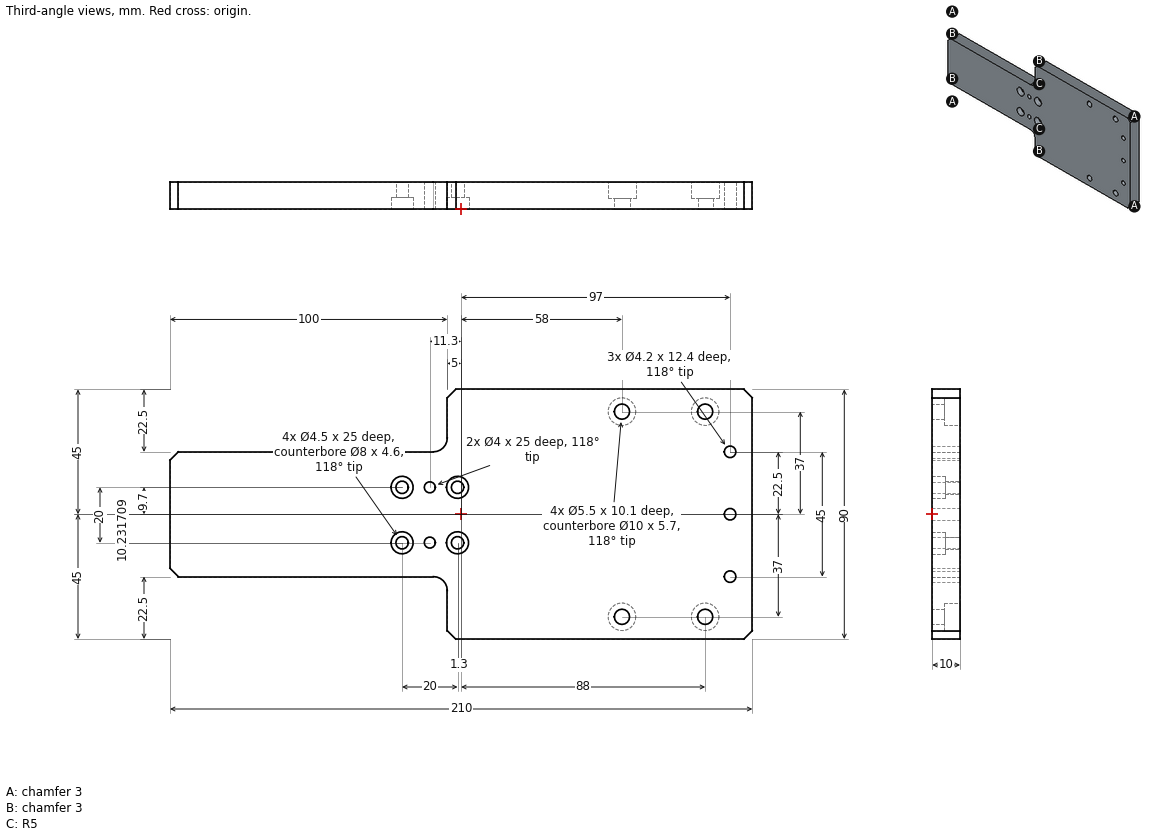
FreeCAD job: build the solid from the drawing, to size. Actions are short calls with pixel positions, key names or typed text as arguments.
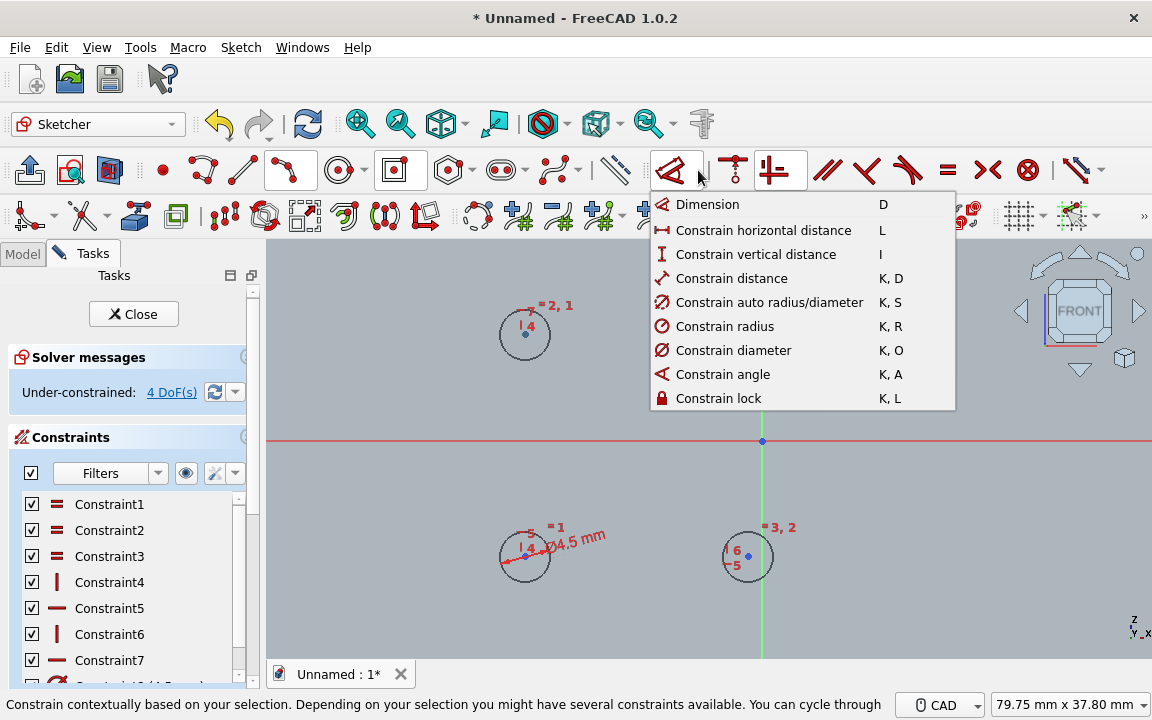
click(803, 254)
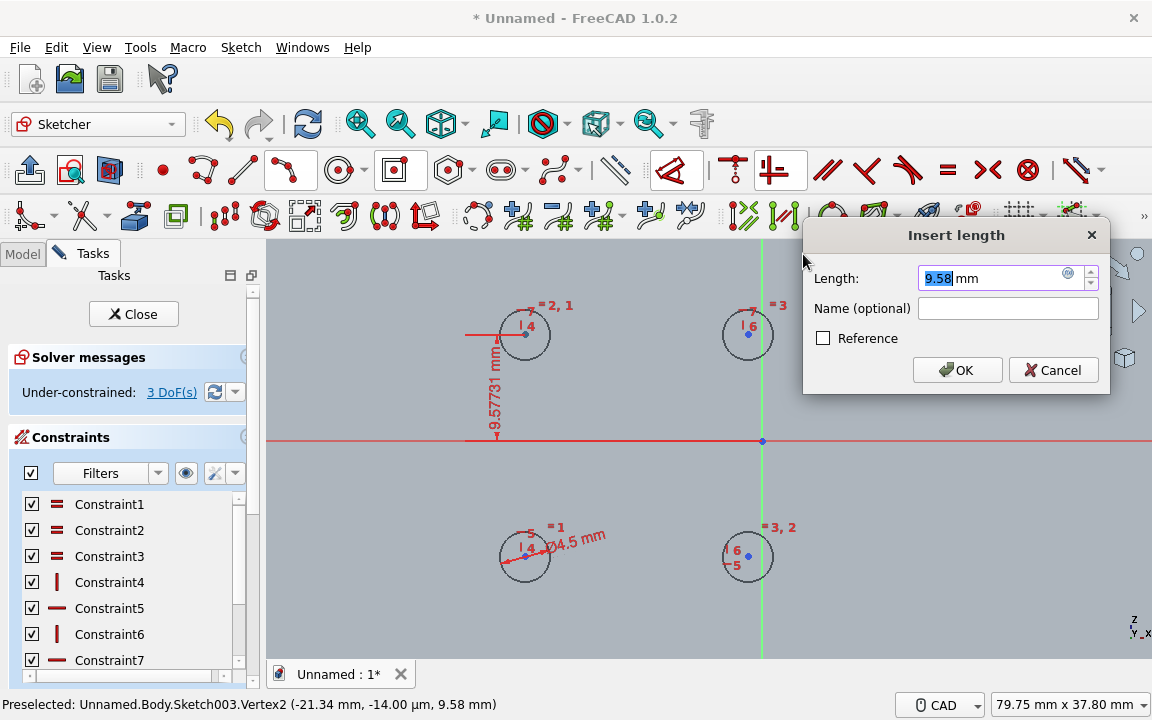
text(9.7)
key(Return)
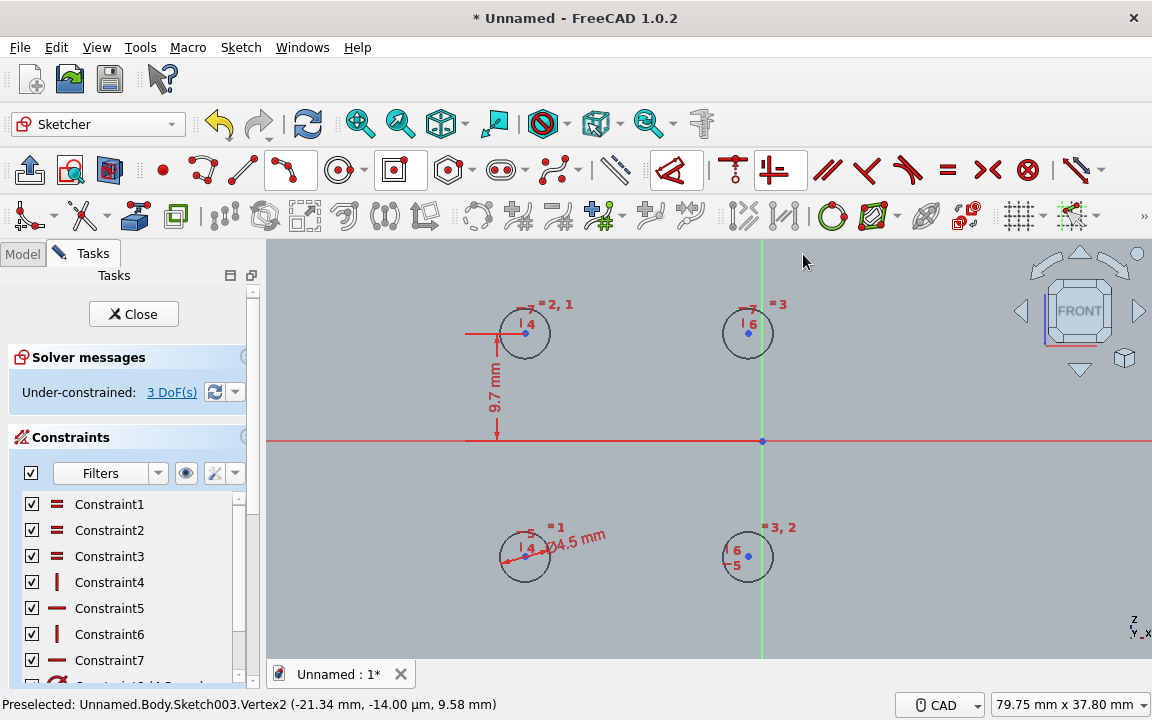
scroll(748, 557, up, 6)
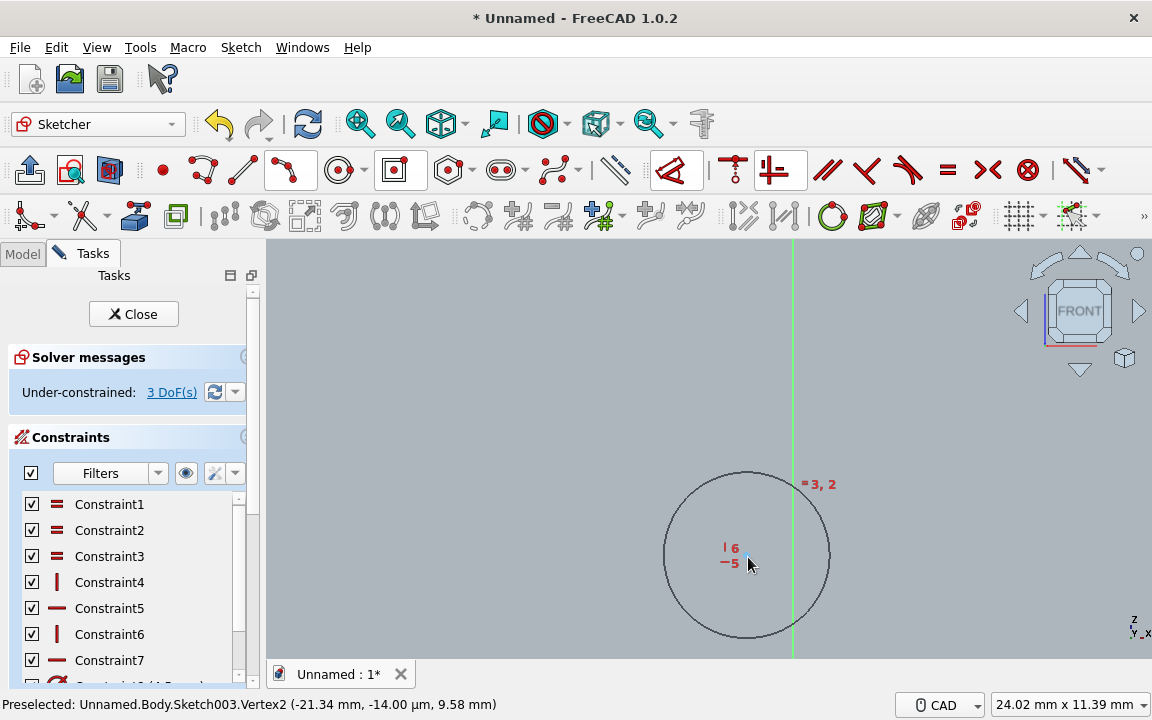
click(747, 555)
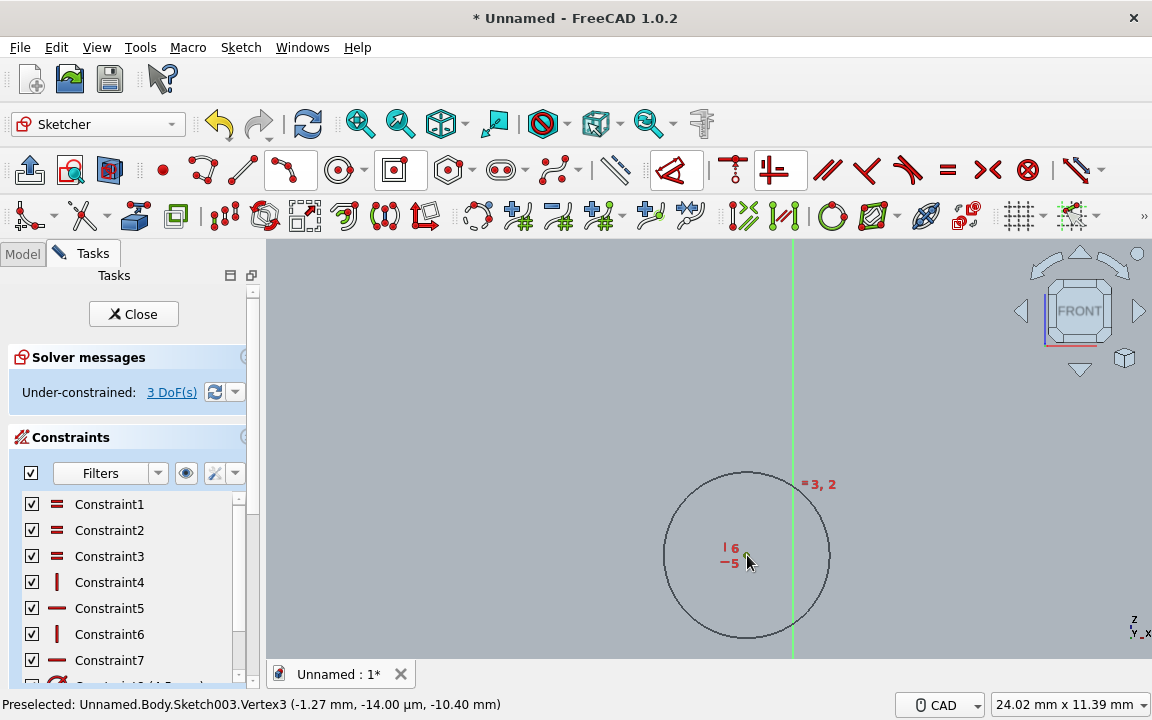
click(698, 170)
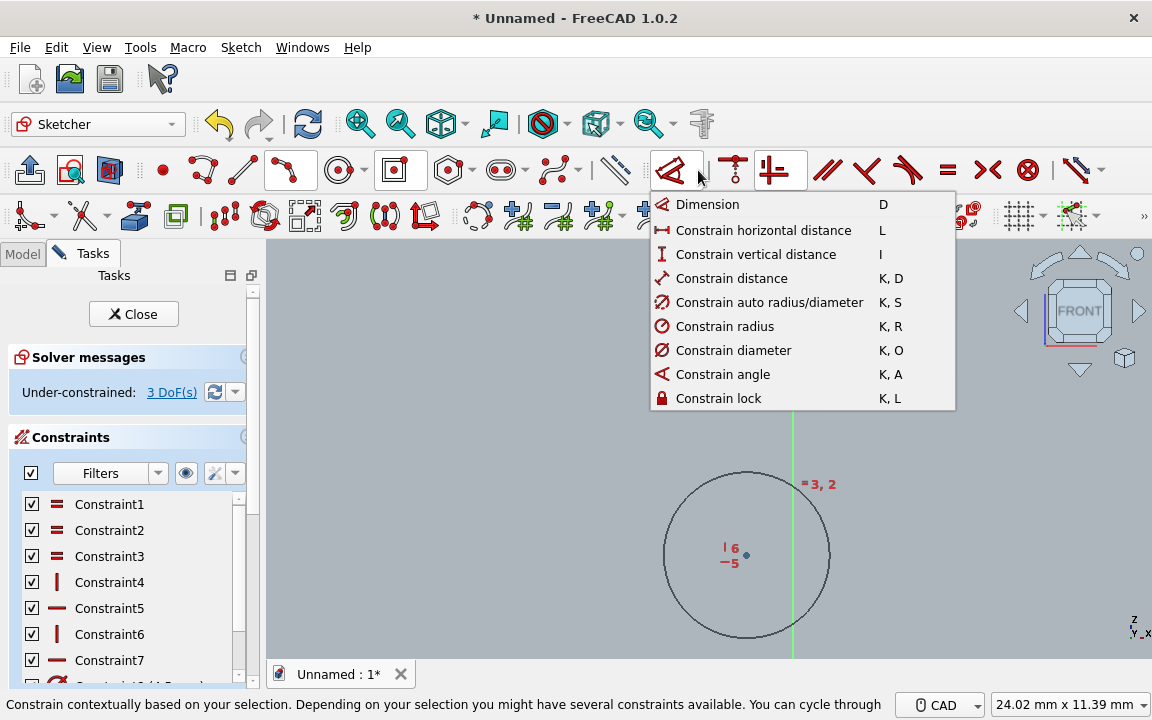
click(803, 230)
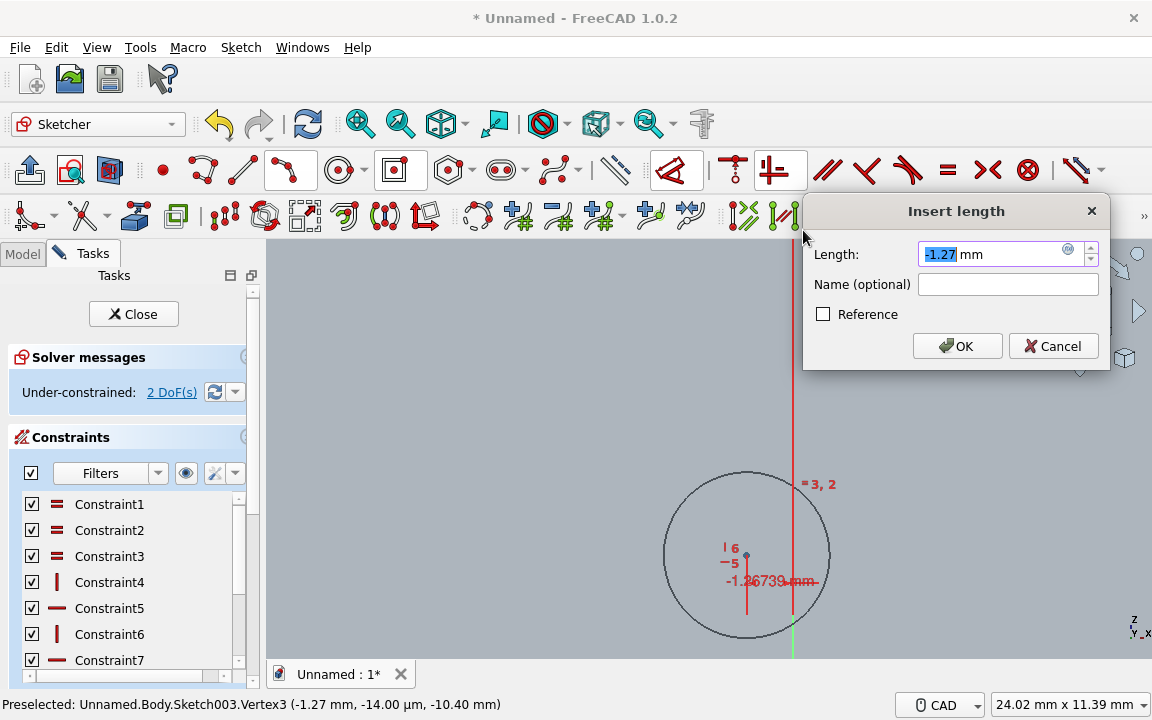
text(-1.3)
key(Return)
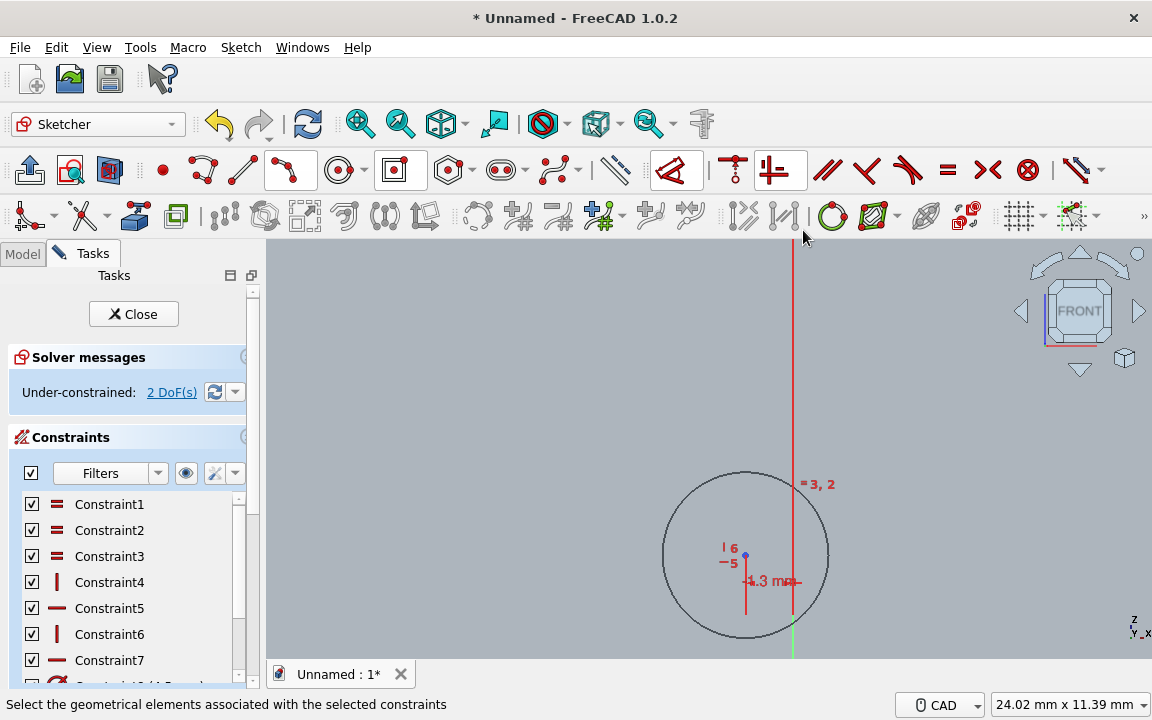
scroll(754, 564, down, 6)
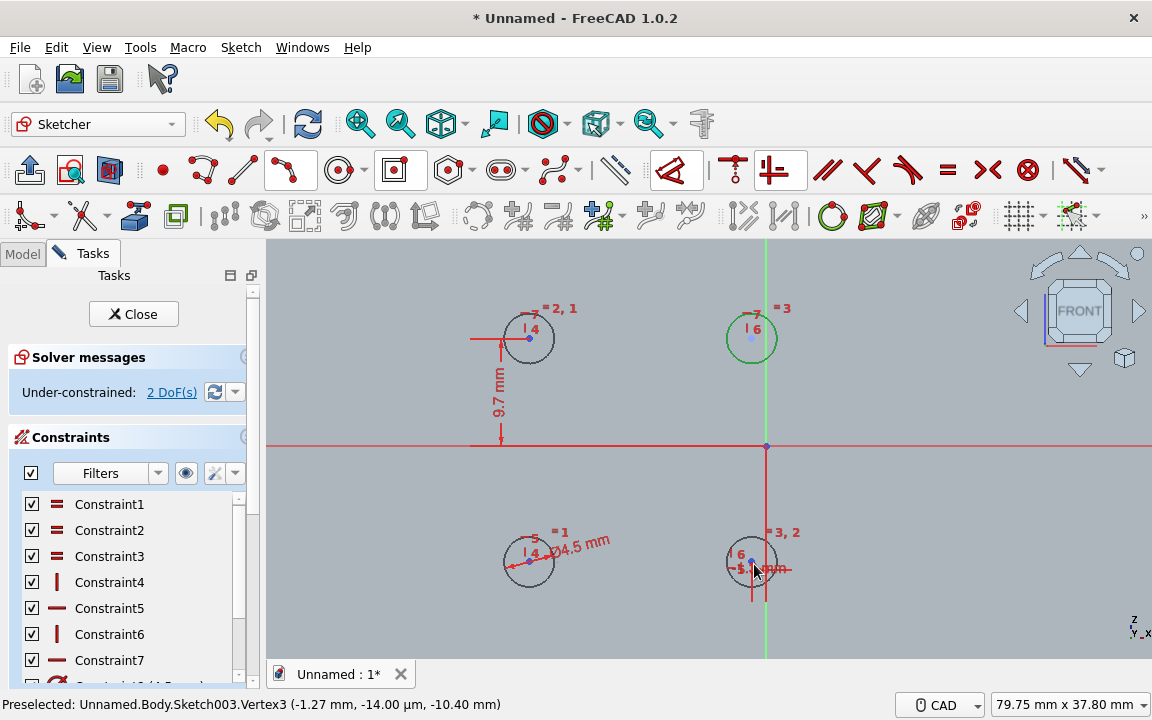
click(529, 562)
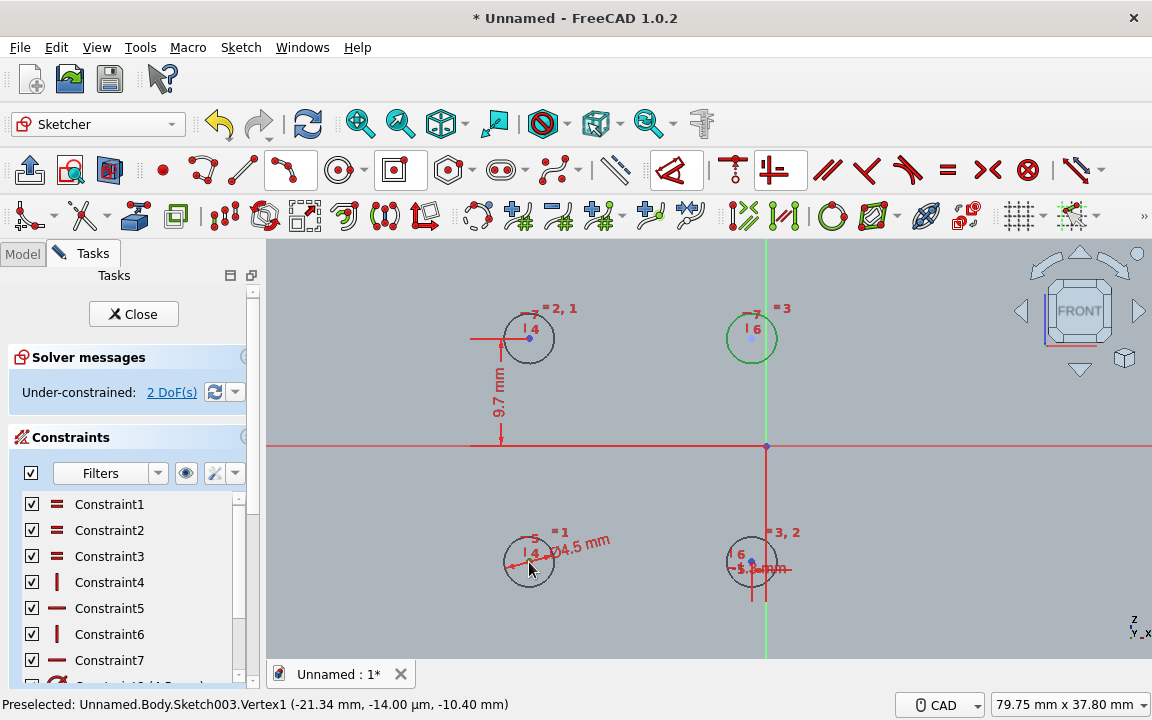
click(529, 339)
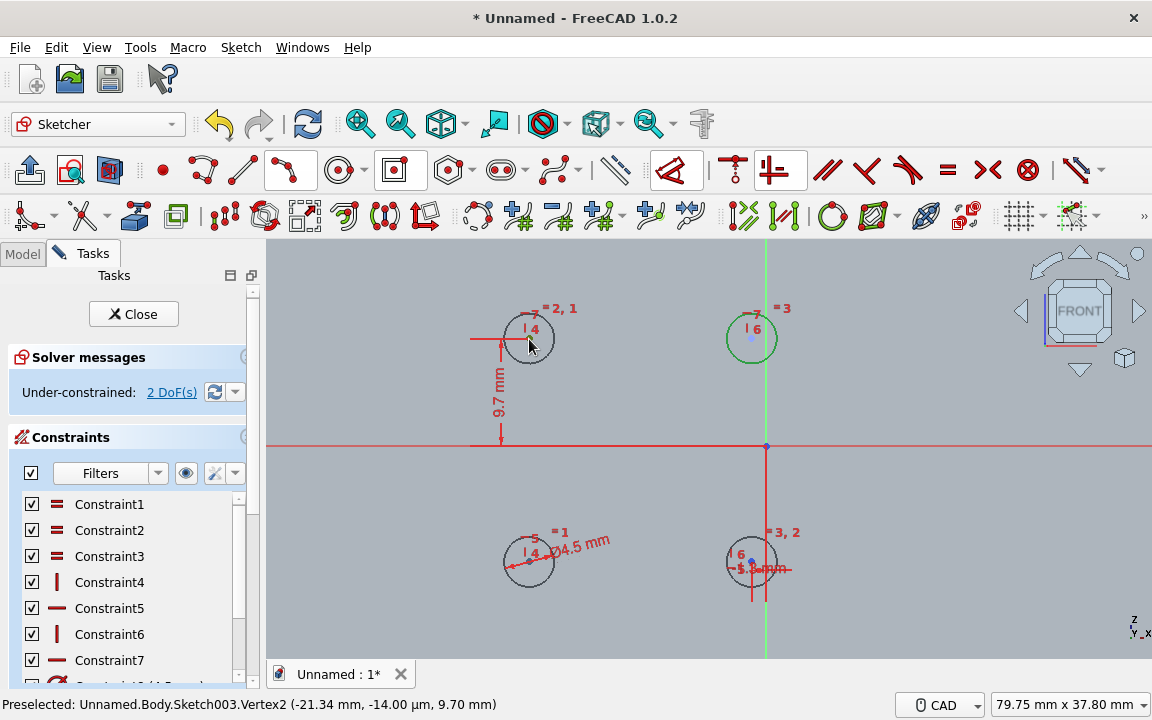
key(i)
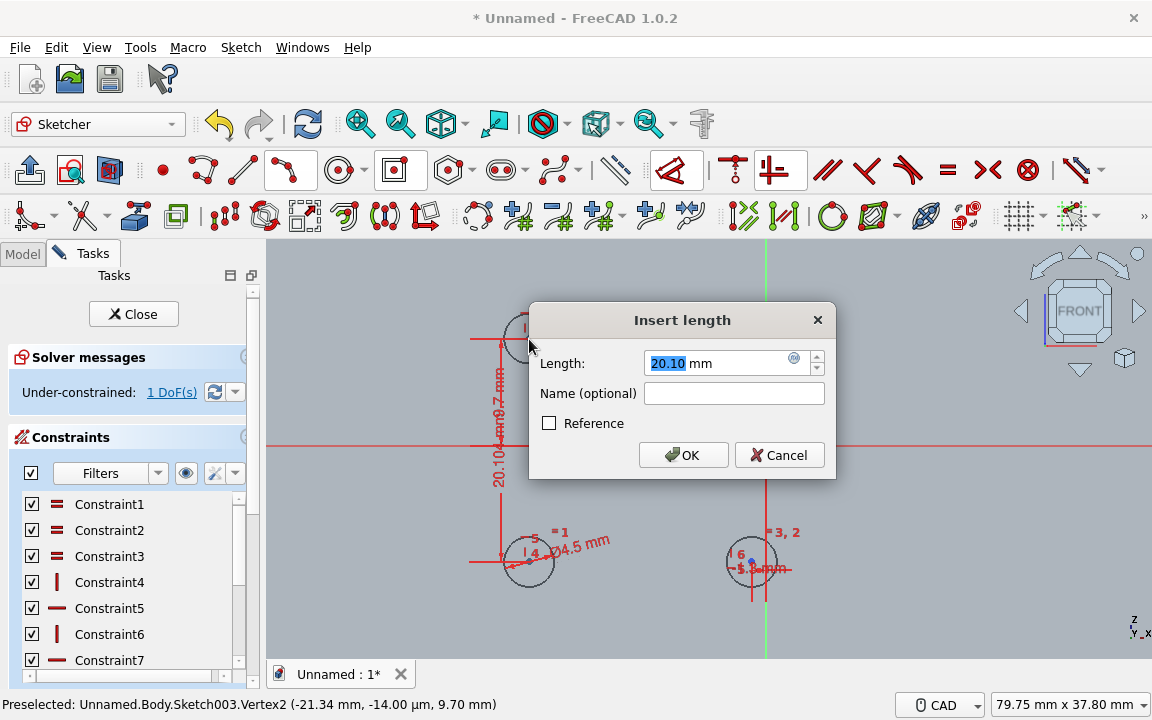
text(20)
key(Return)